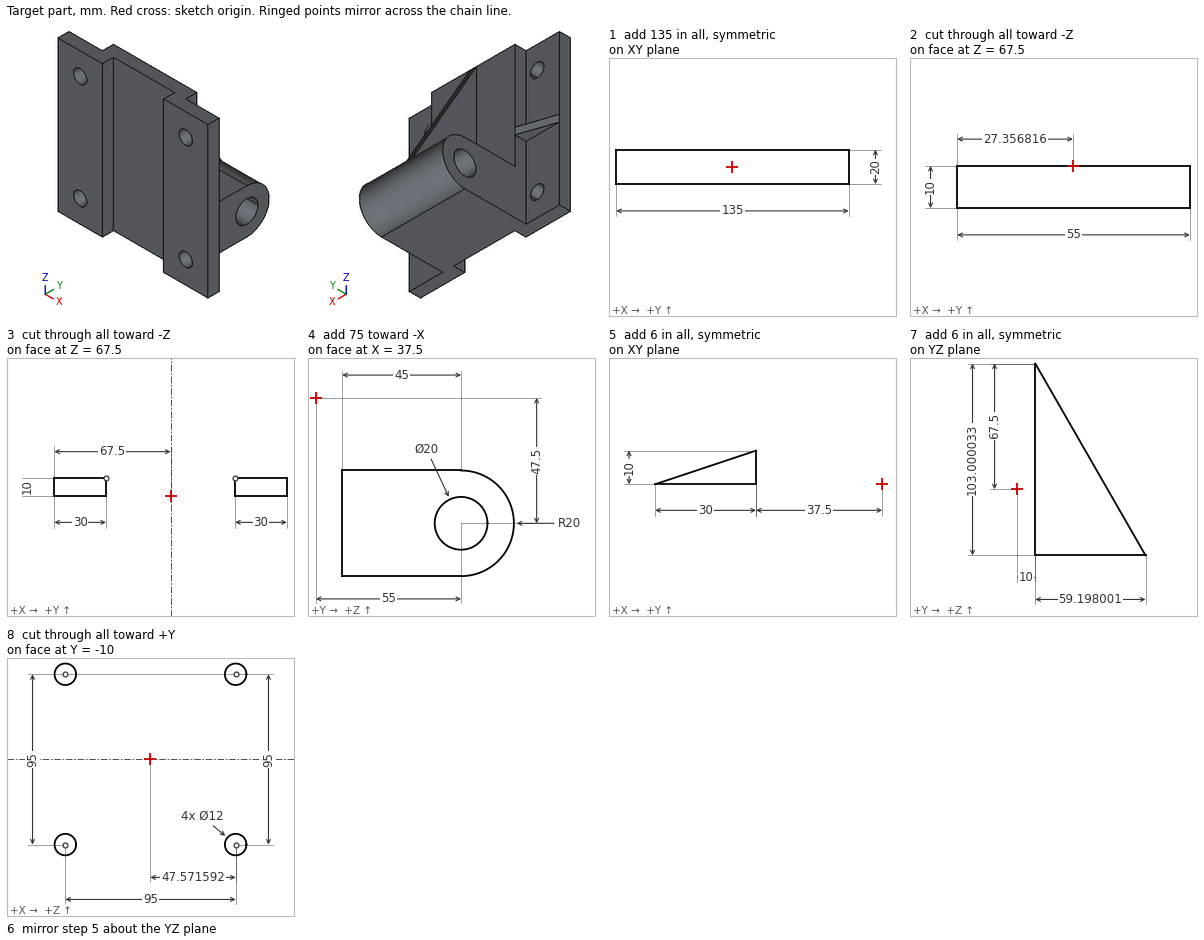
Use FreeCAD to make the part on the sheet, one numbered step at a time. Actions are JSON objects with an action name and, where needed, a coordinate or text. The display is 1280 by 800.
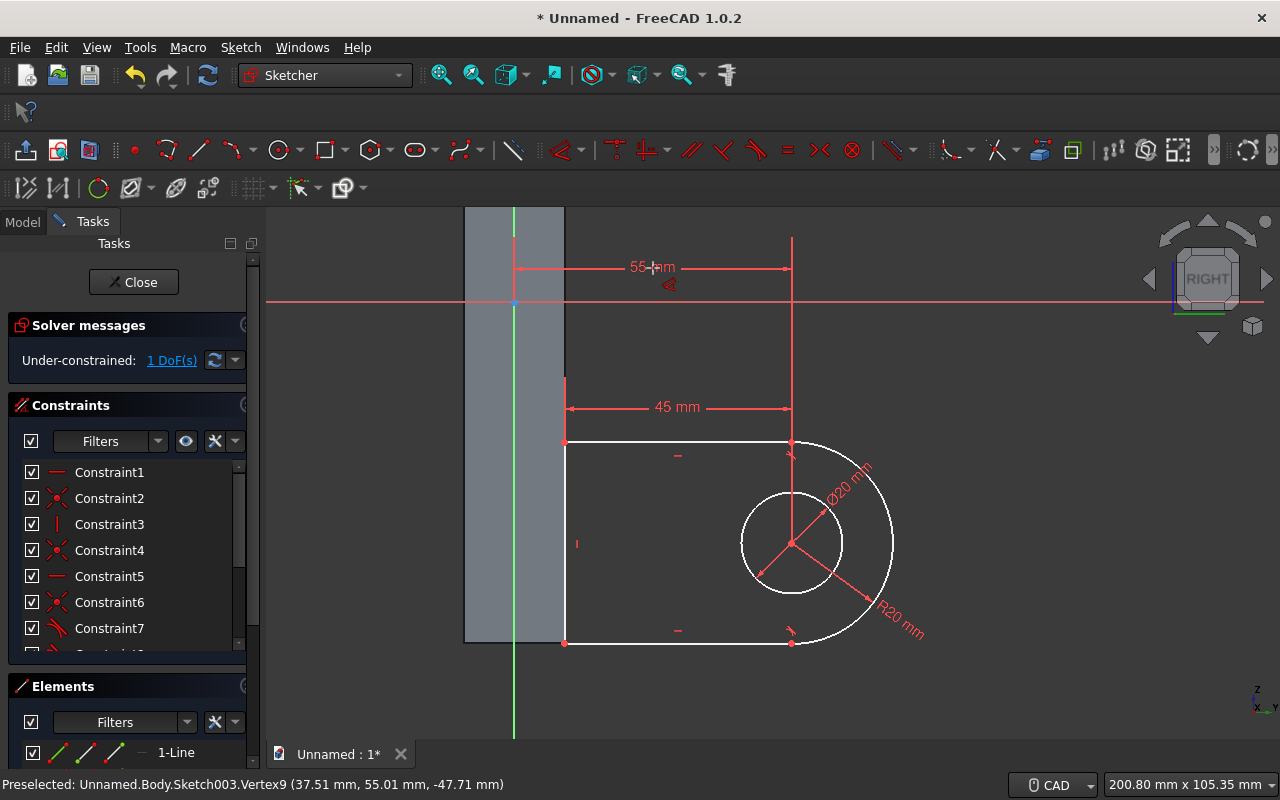
{"action": "left_click", "coordinate": [792, 543]}
{"action": "left_click", "coordinate": [480, 423]}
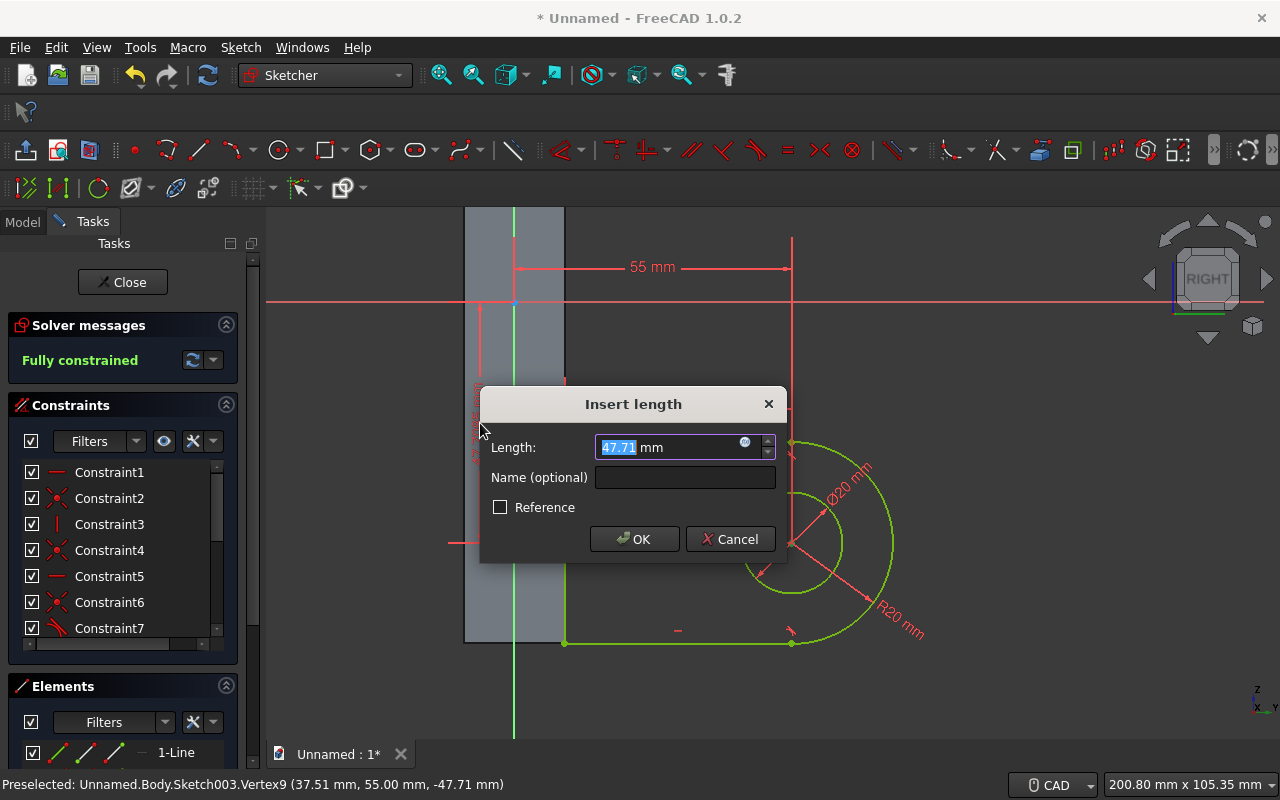
{"action": "type", "text": "47.5"}
{"action": "key", "text": "Return"}
{"action": "key", "text": "Escape"}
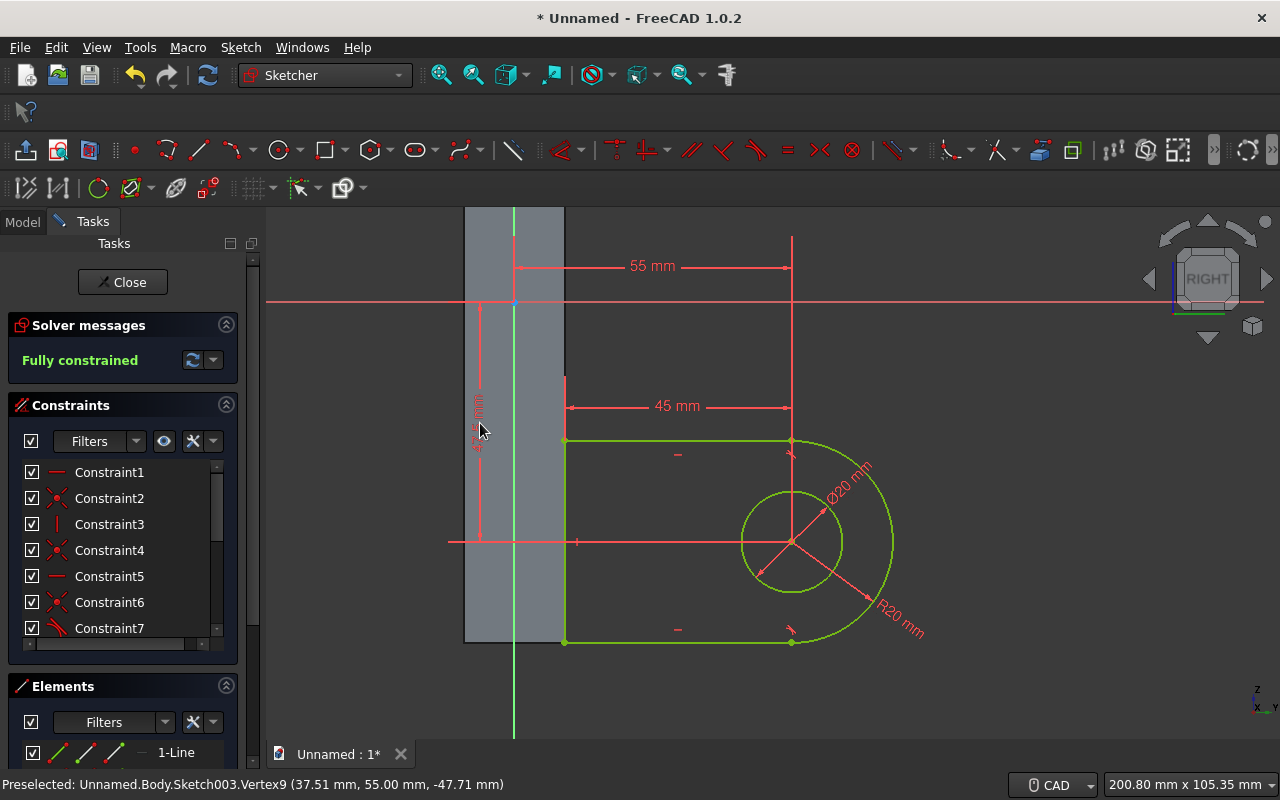
{"action": "left_click", "coordinate": [123, 282]}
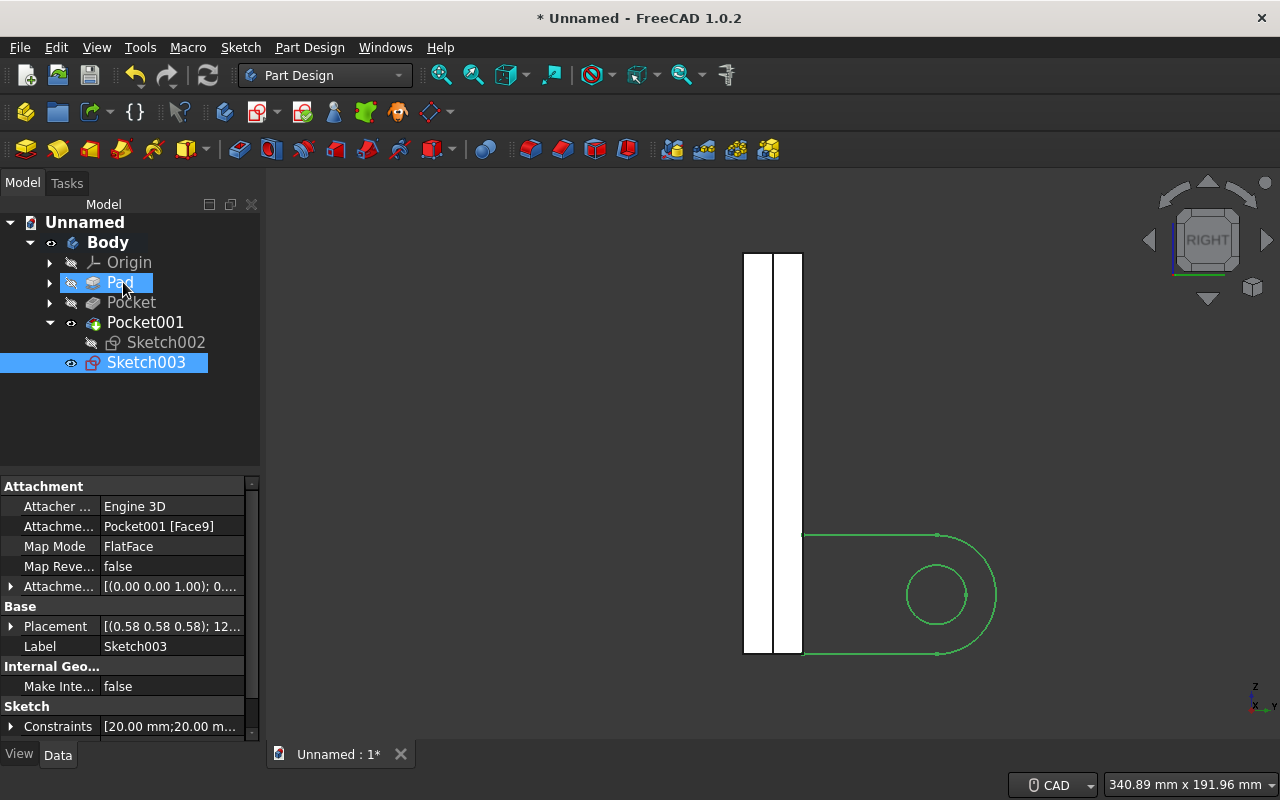
{"action": "left_click", "coordinate": [26, 150]}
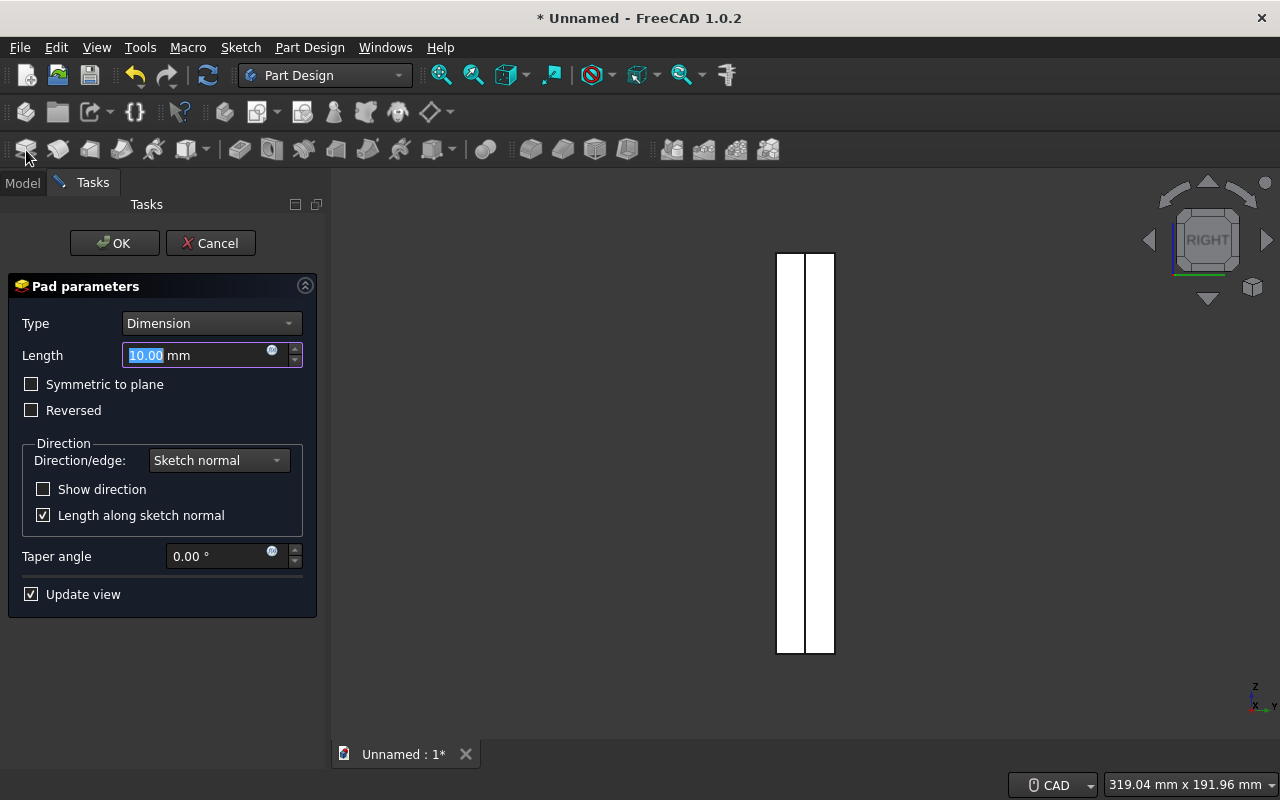
{"action": "type", "text": "75"}
{"action": "key", "text": "Tab"}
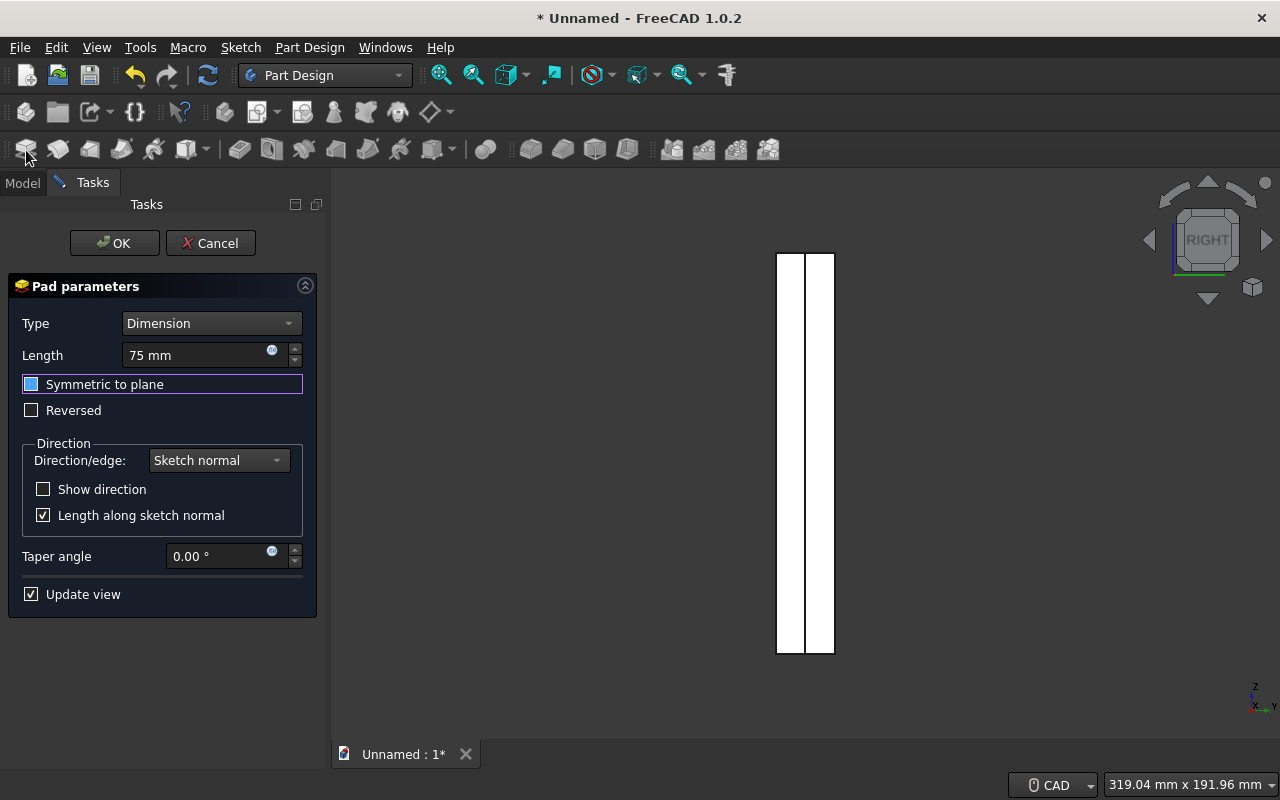
{"action": "left_click", "coordinate": [30, 410]}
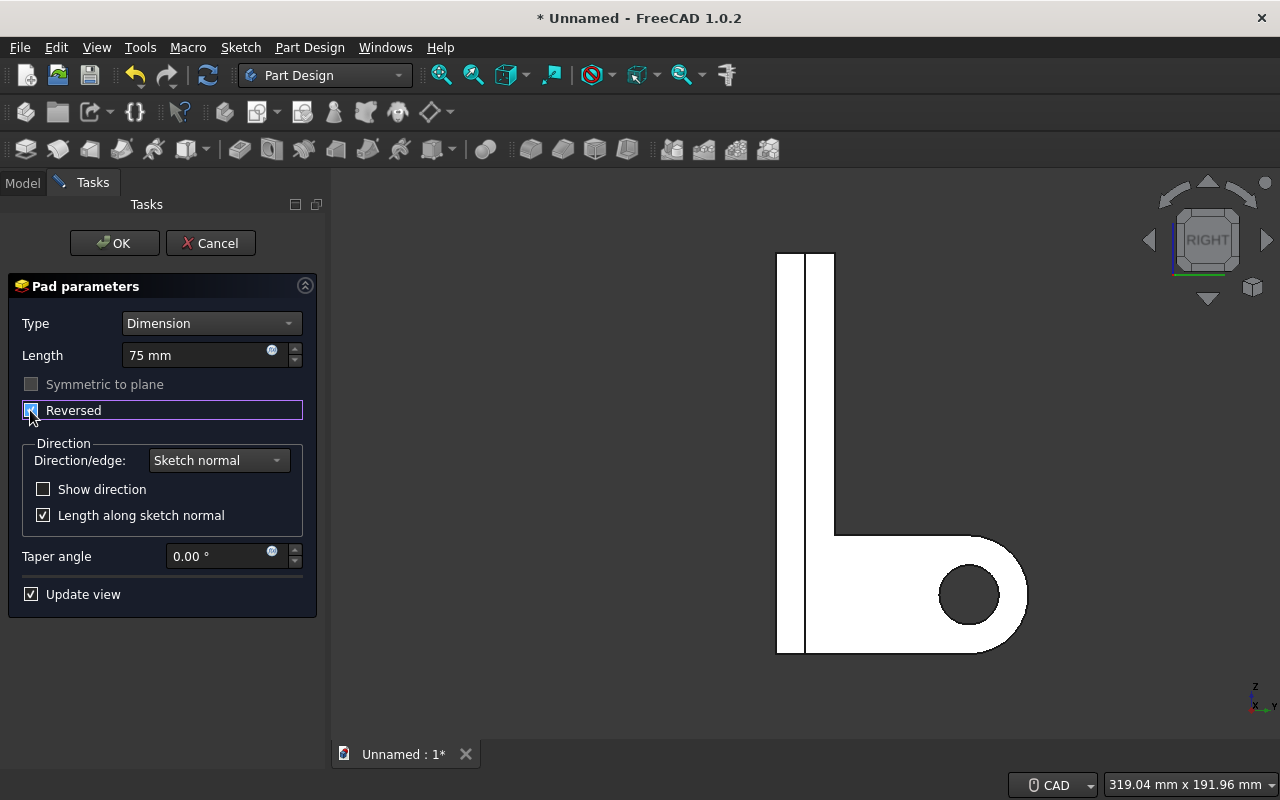
{"action": "left_click", "coordinate": [115, 243]}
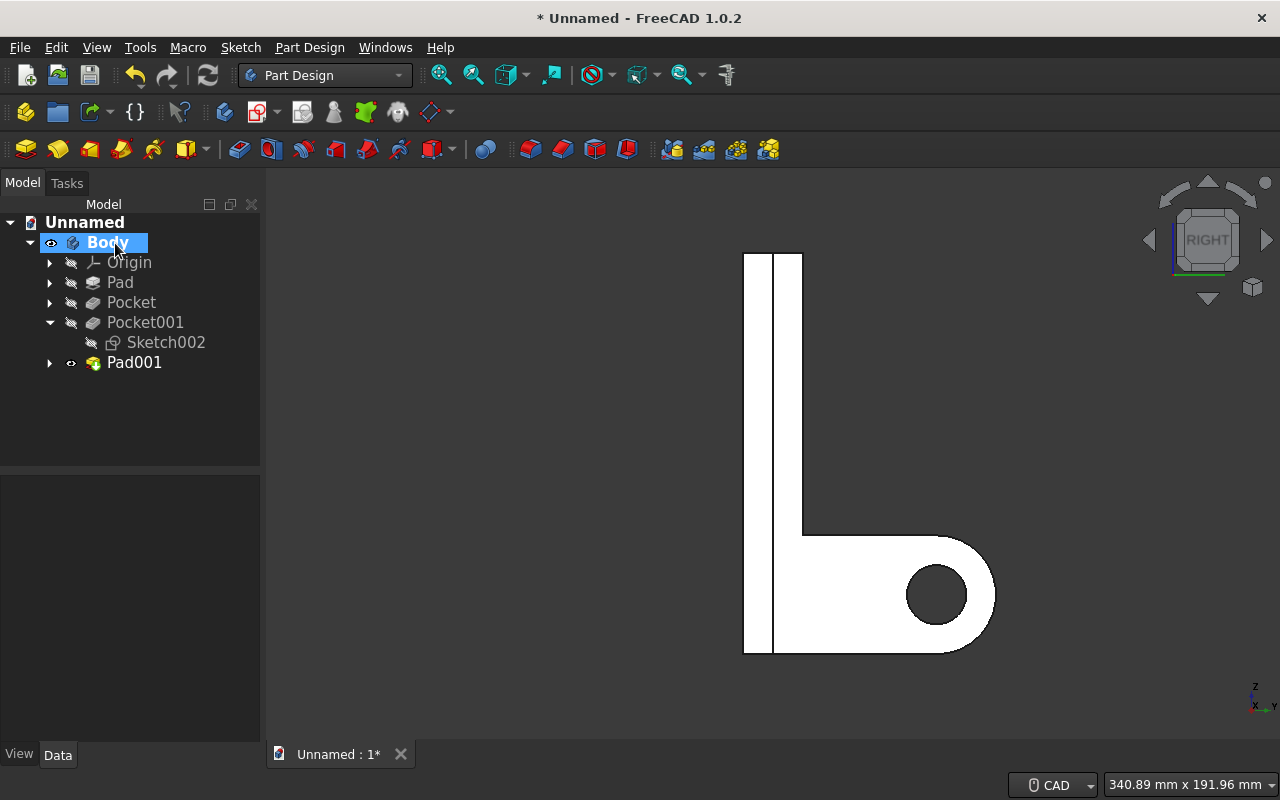
{"action": "left_click", "coordinate": [258, 112]}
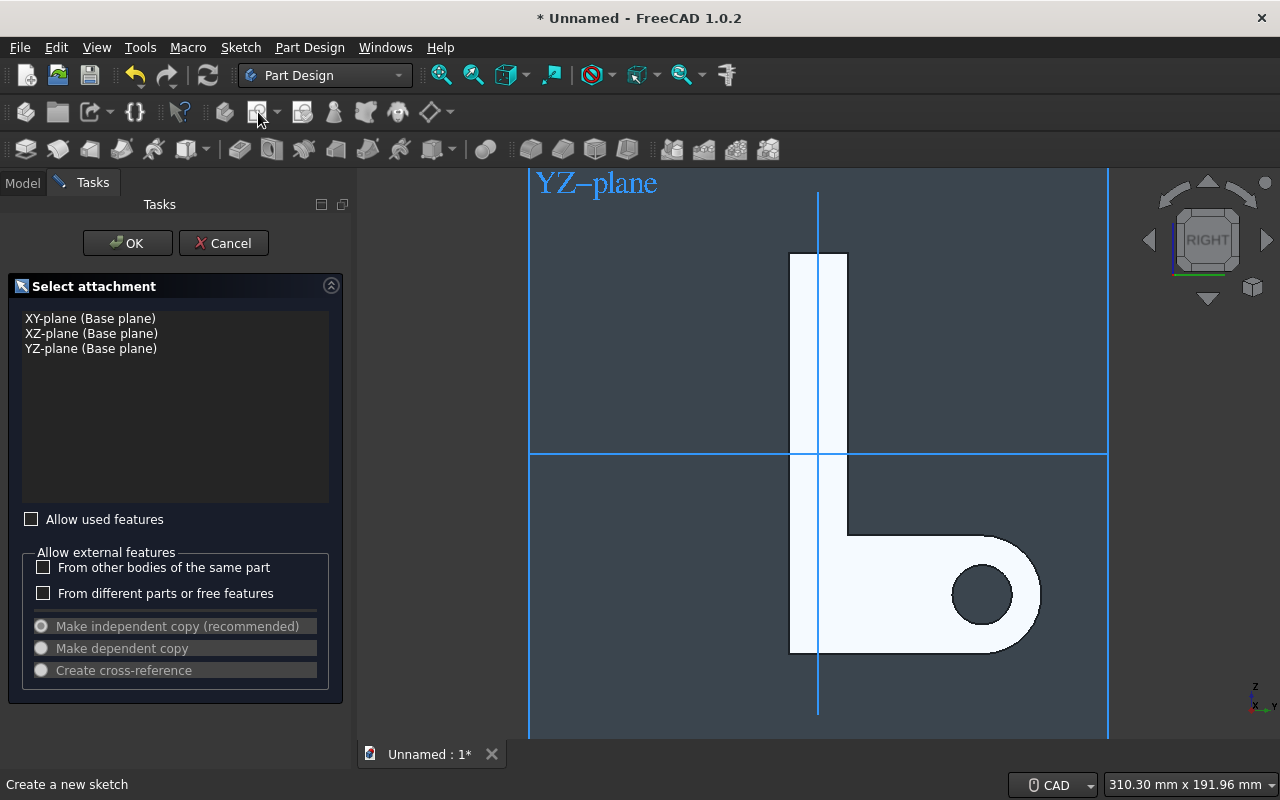
{"action": "left_click", "coordinate": [82, 318]}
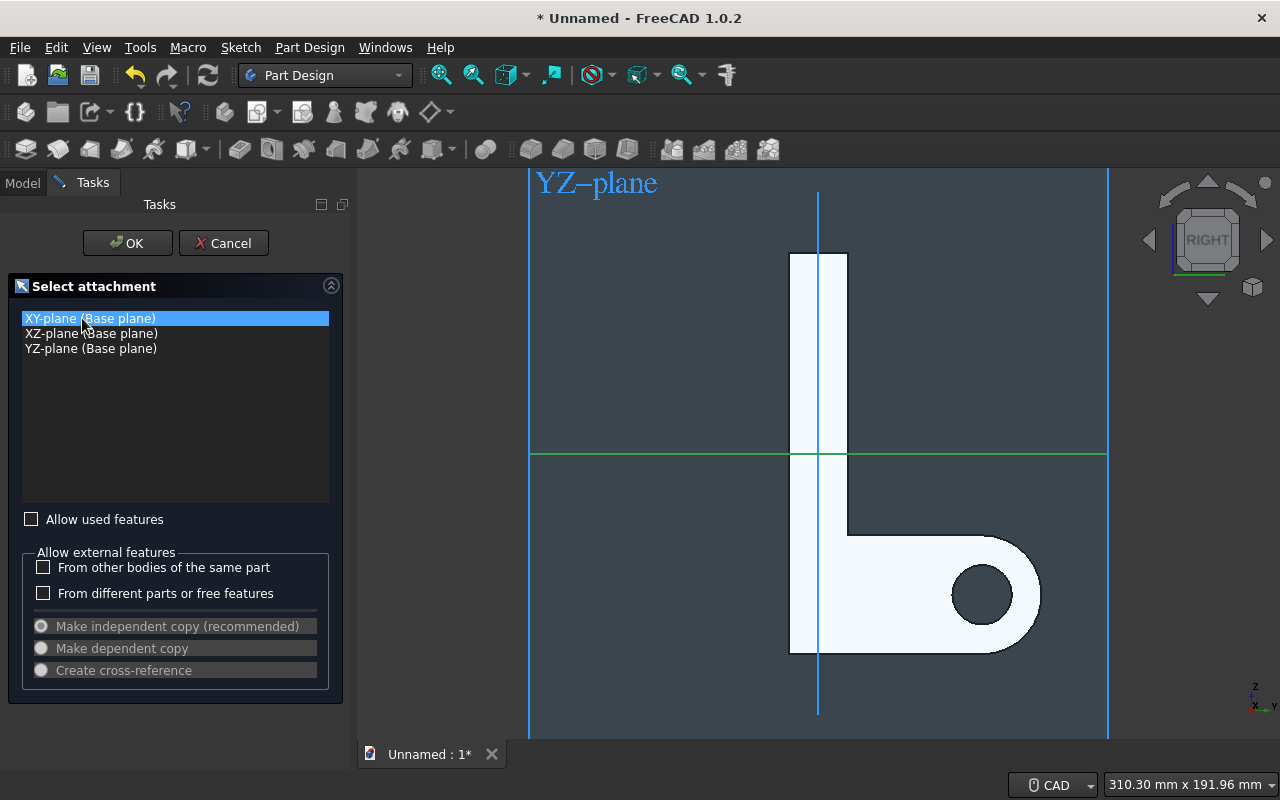
{"action": "left_click", "coordinate": [128, 243]}